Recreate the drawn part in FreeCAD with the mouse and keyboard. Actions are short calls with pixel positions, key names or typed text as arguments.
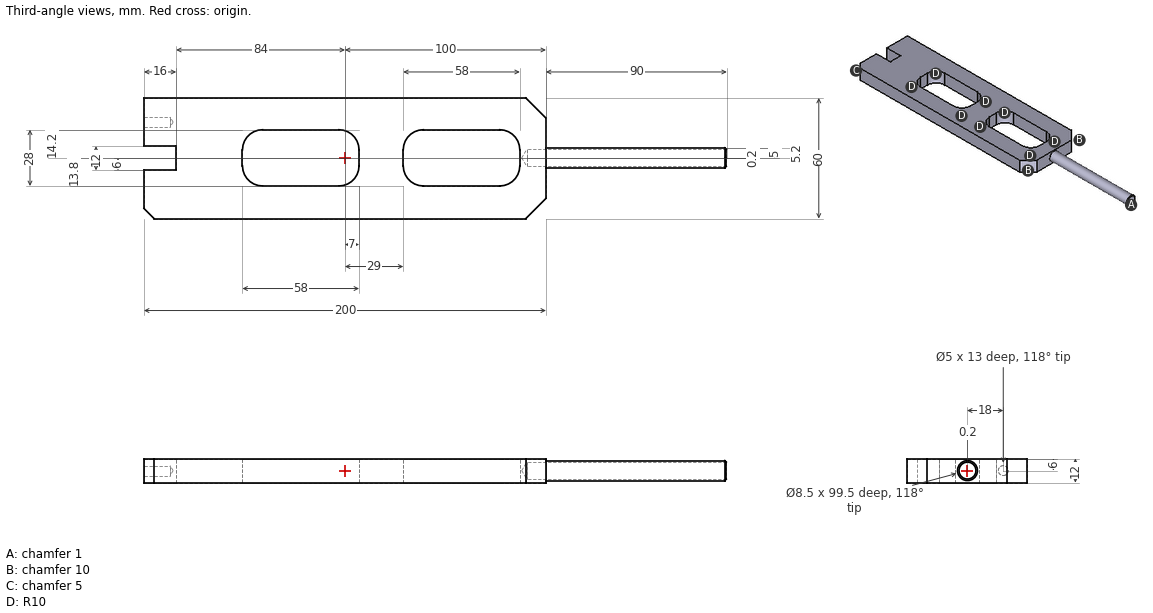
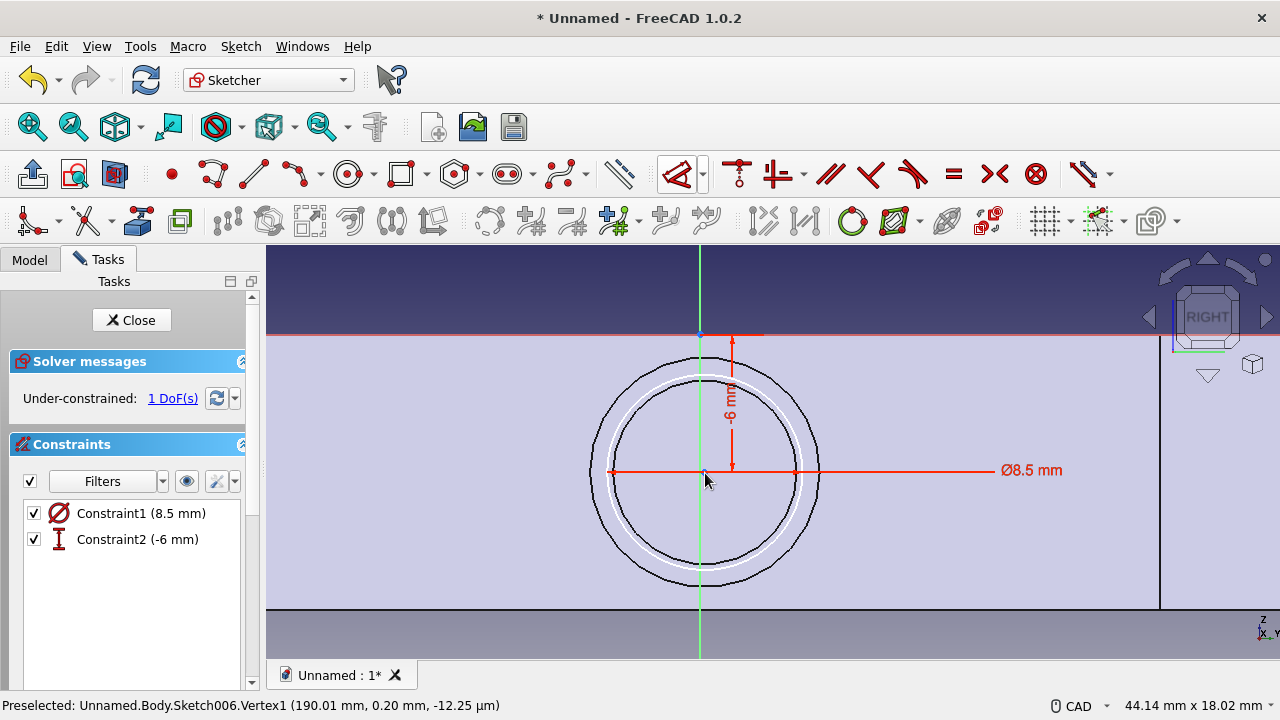
scroll(705, 472, up, 11)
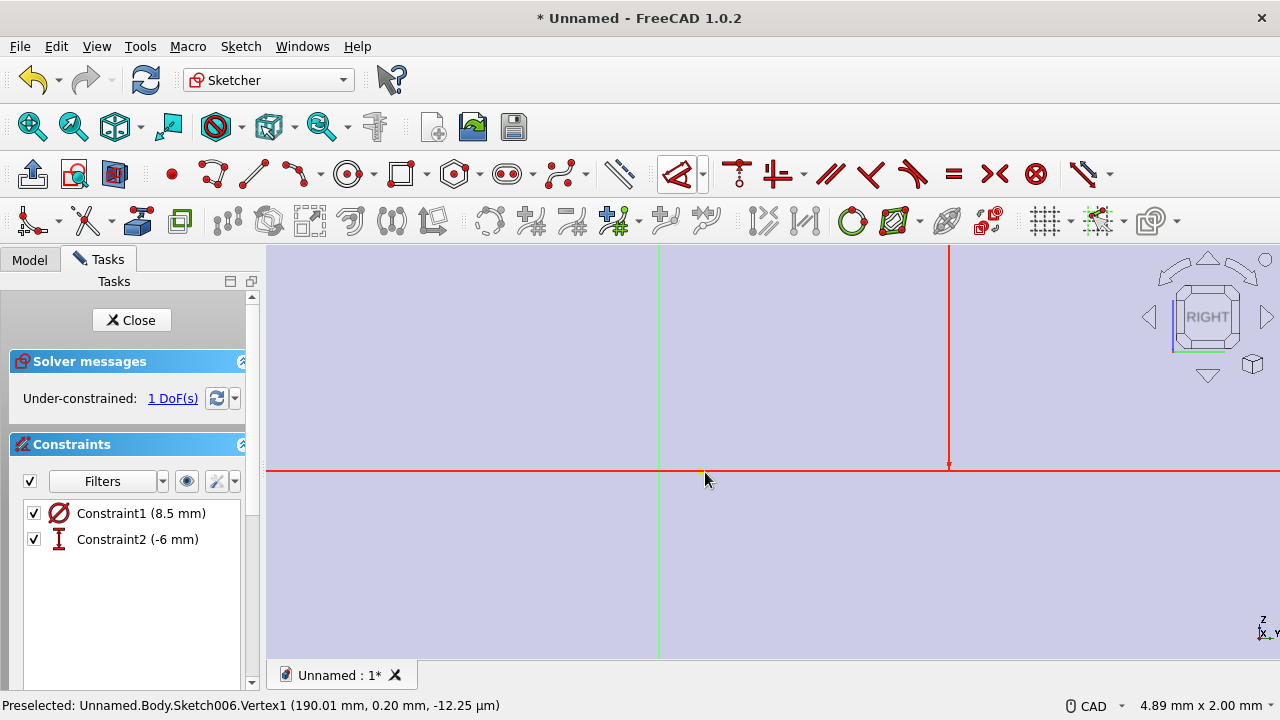
click(700, 471)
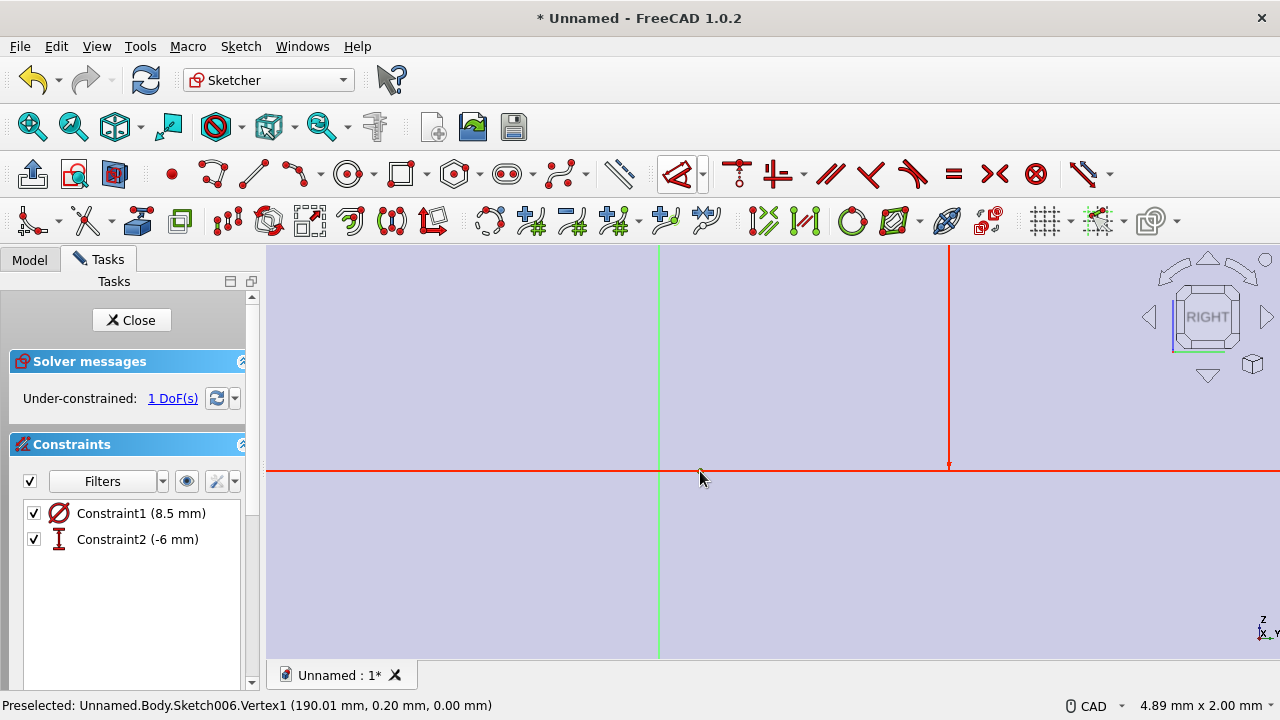
key(l)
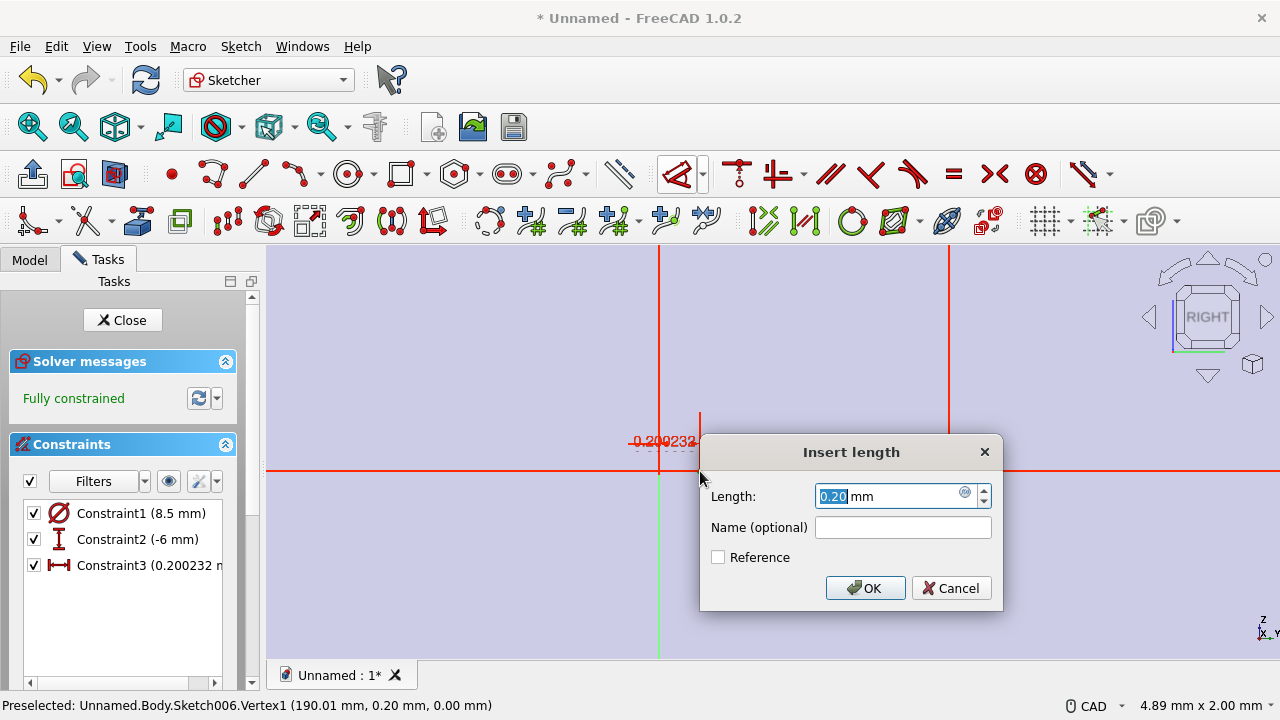
text(0.2)
key(Return)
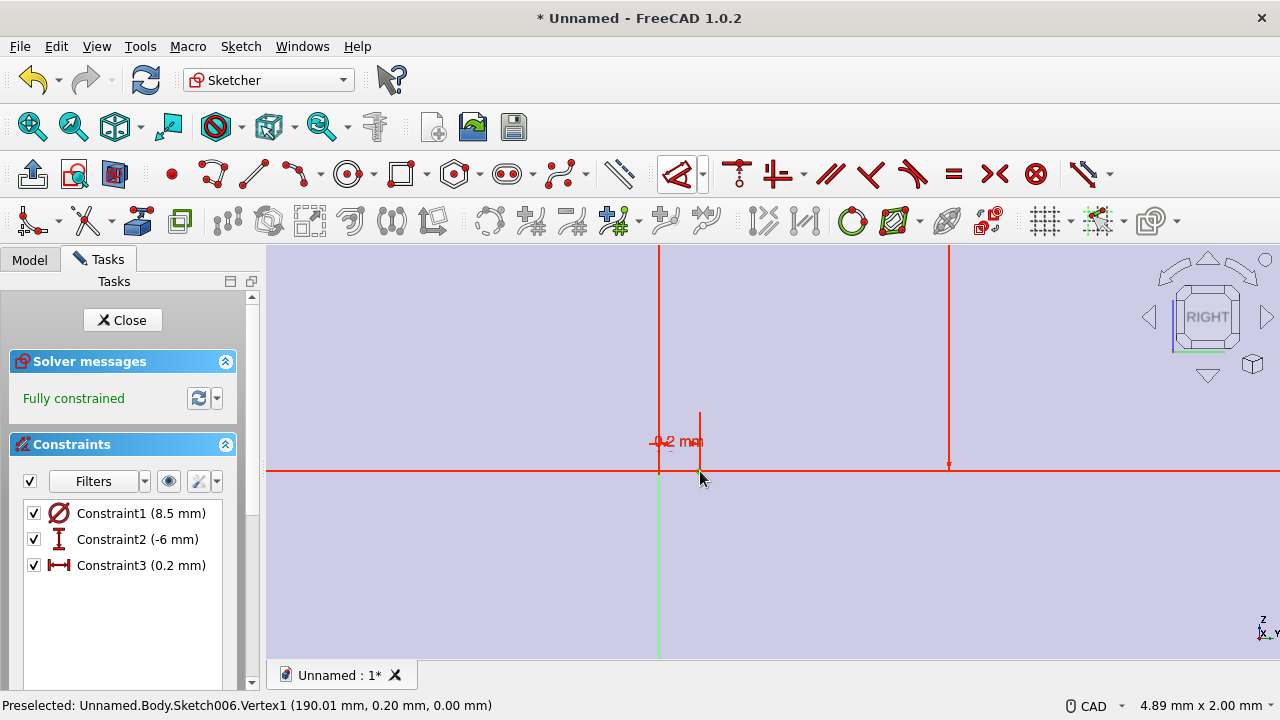
click(123, 320)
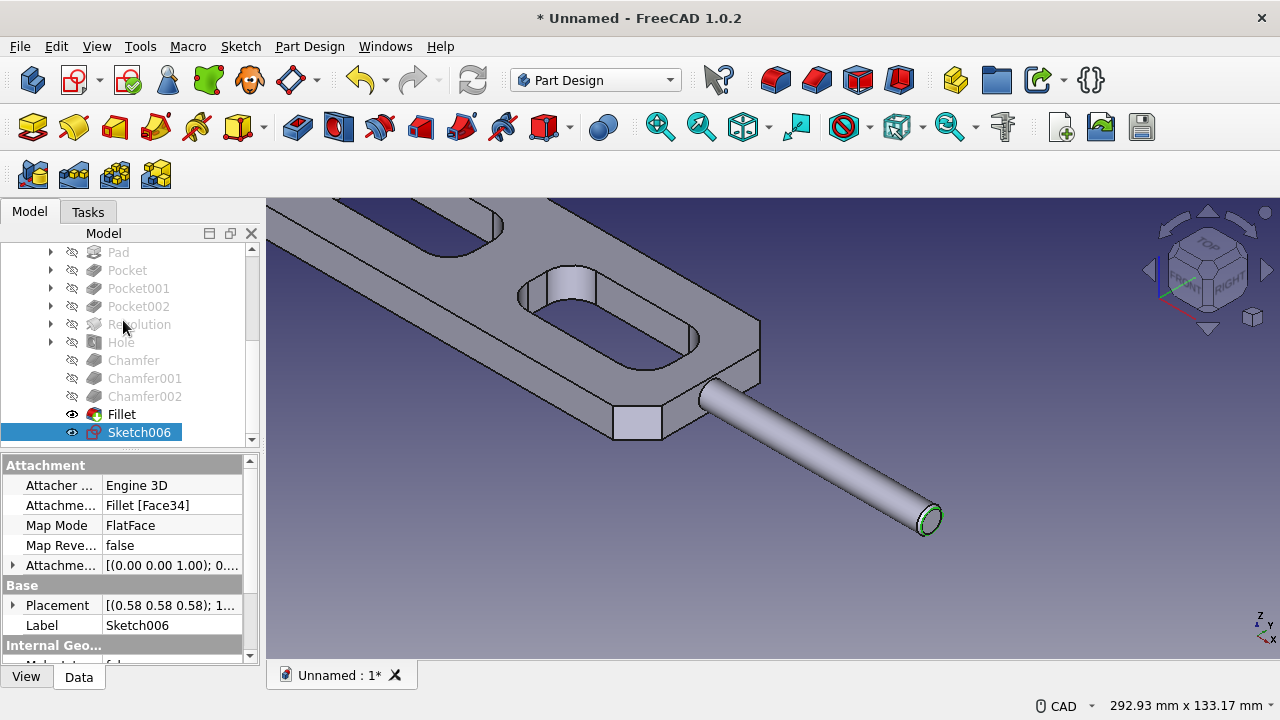
click(339, 128)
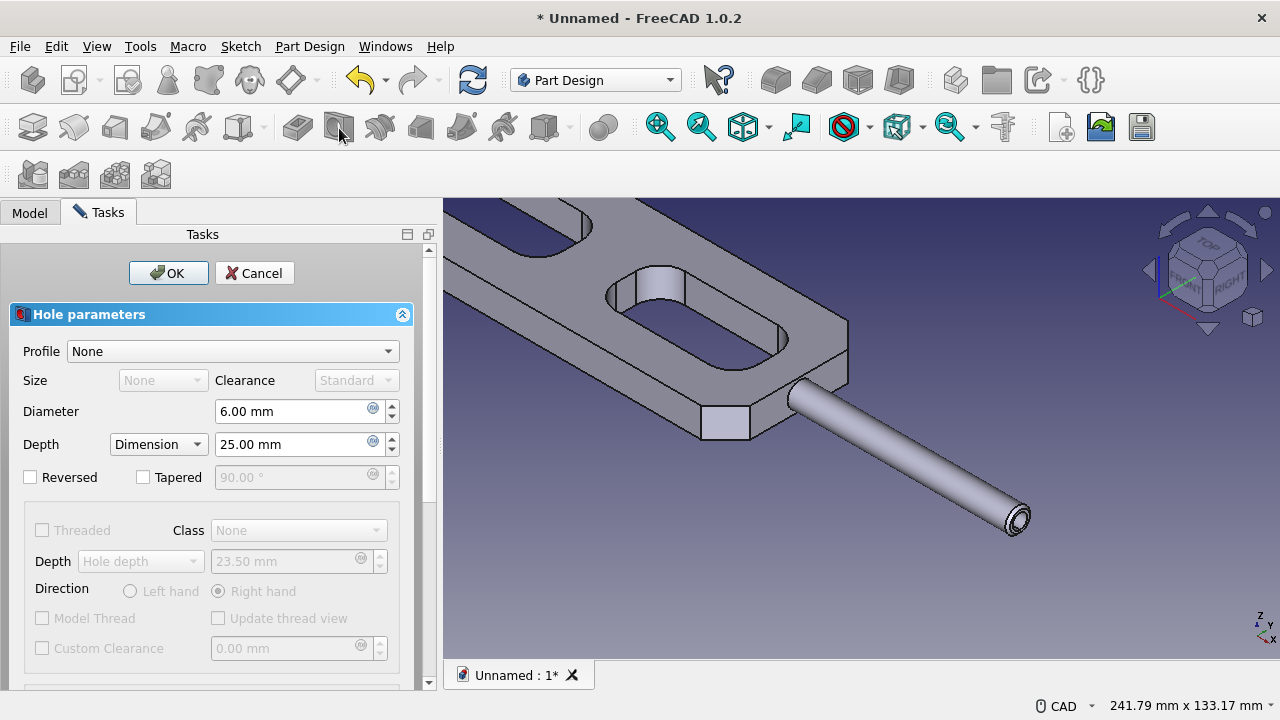
triple_click(300, 412)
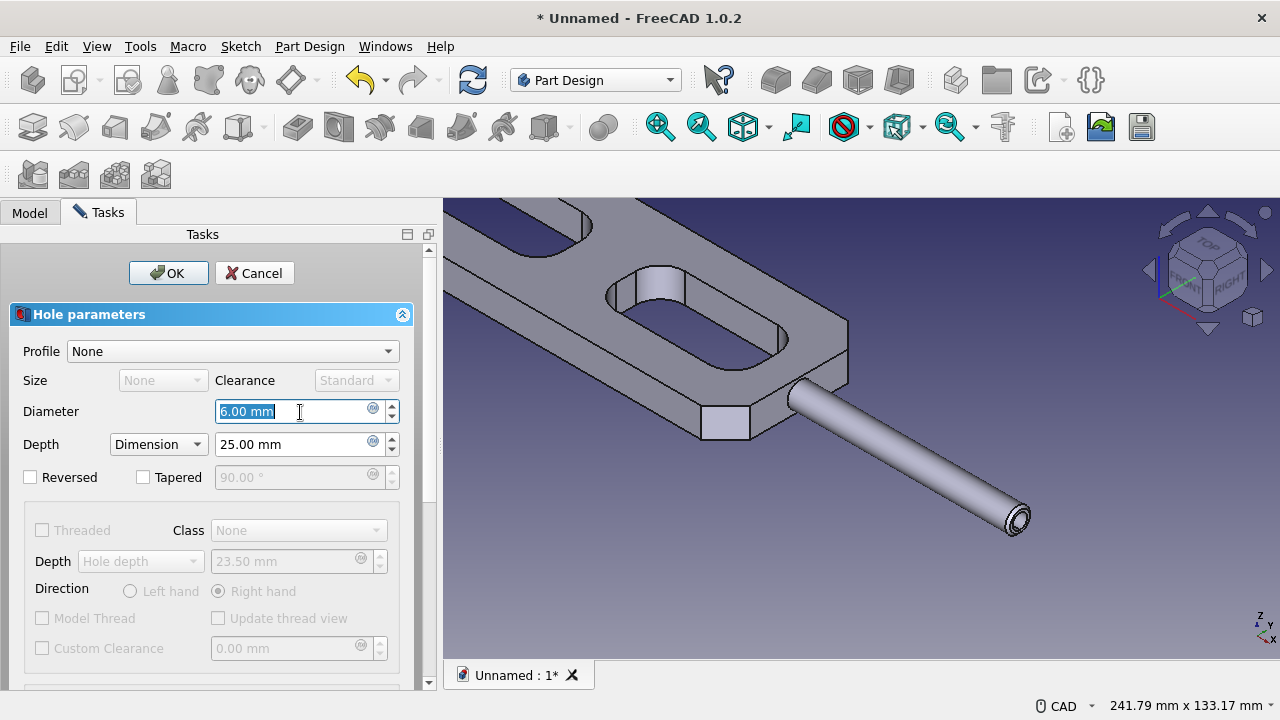
text(8.5)
key(Tab)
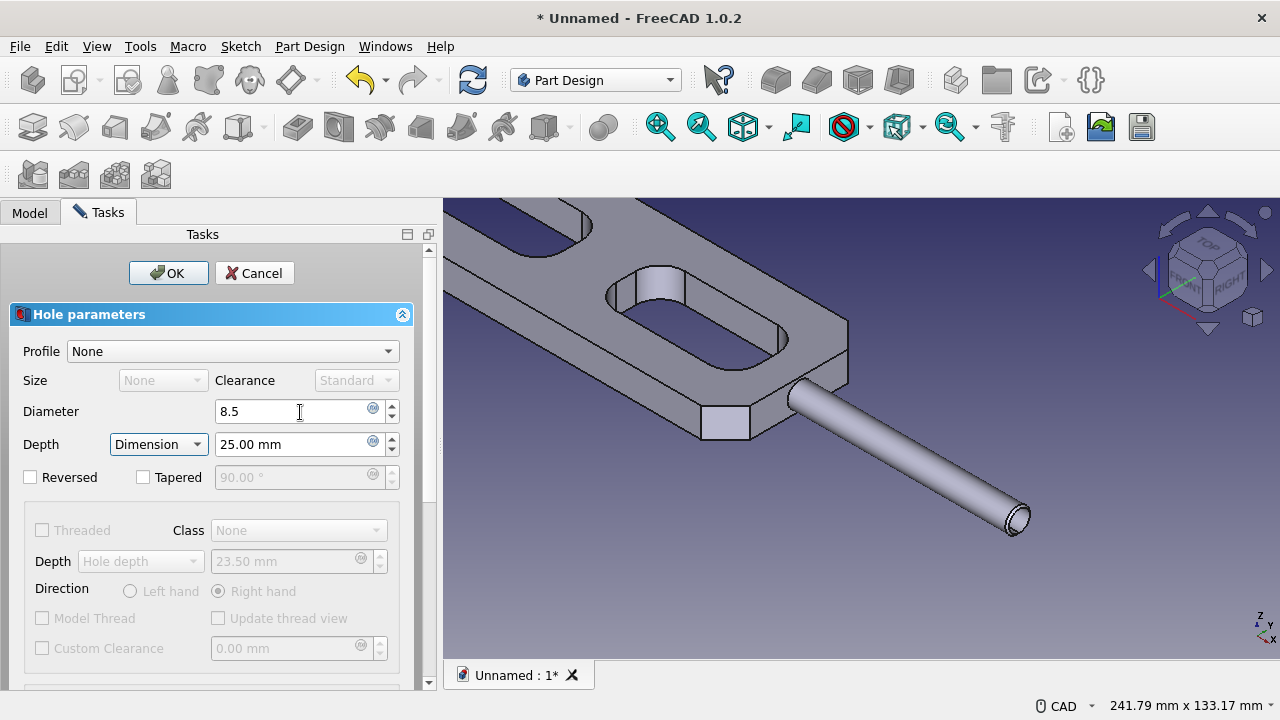
triple_click(300, 444)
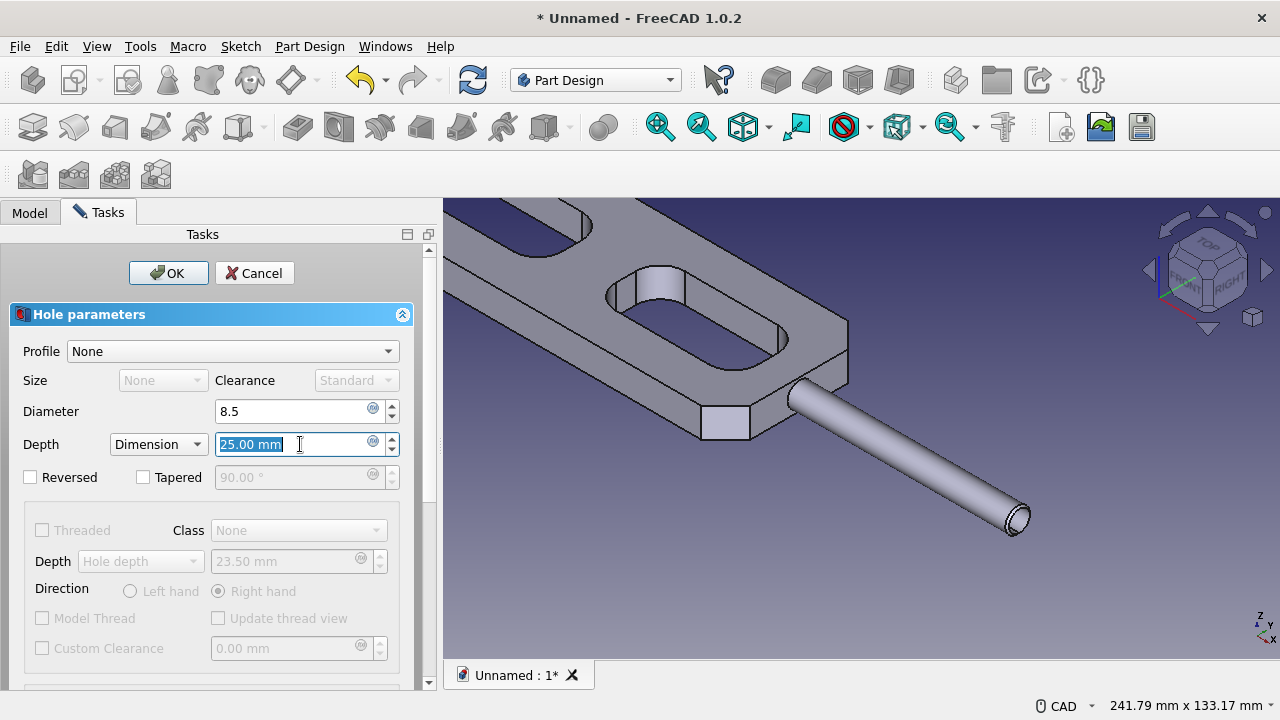
text(99.5)
key(Tab)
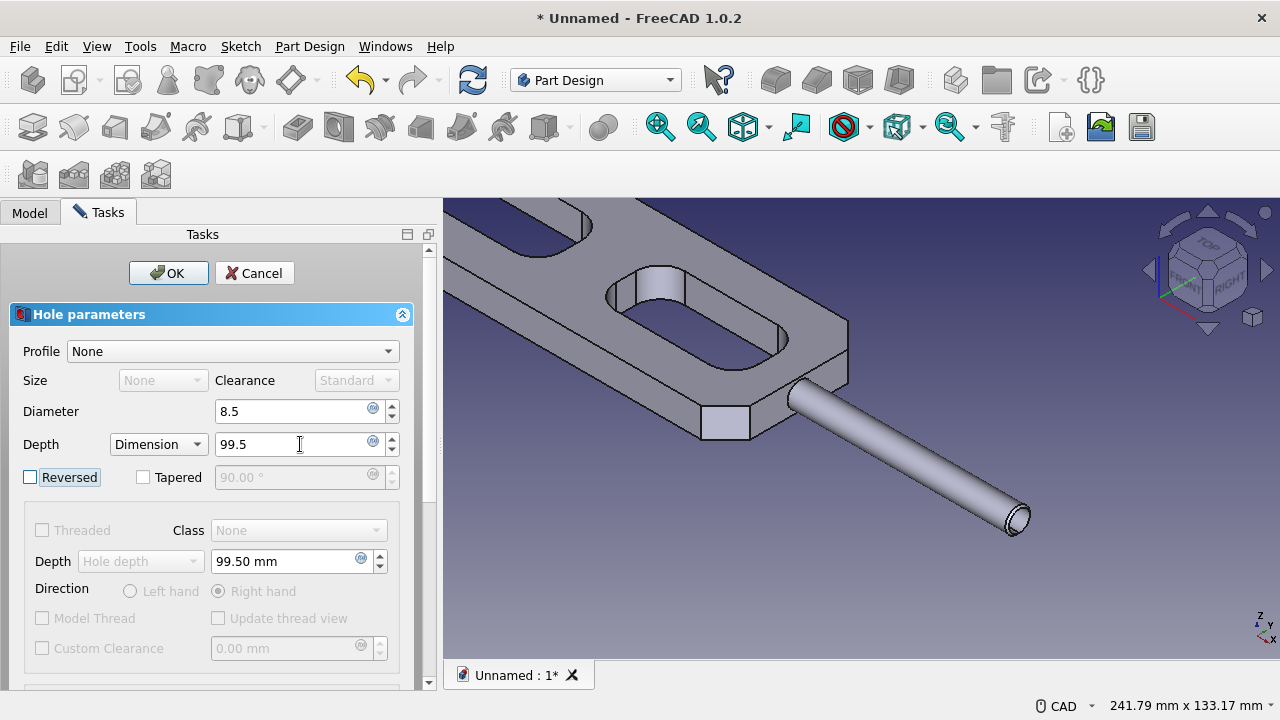
click(169, 273)